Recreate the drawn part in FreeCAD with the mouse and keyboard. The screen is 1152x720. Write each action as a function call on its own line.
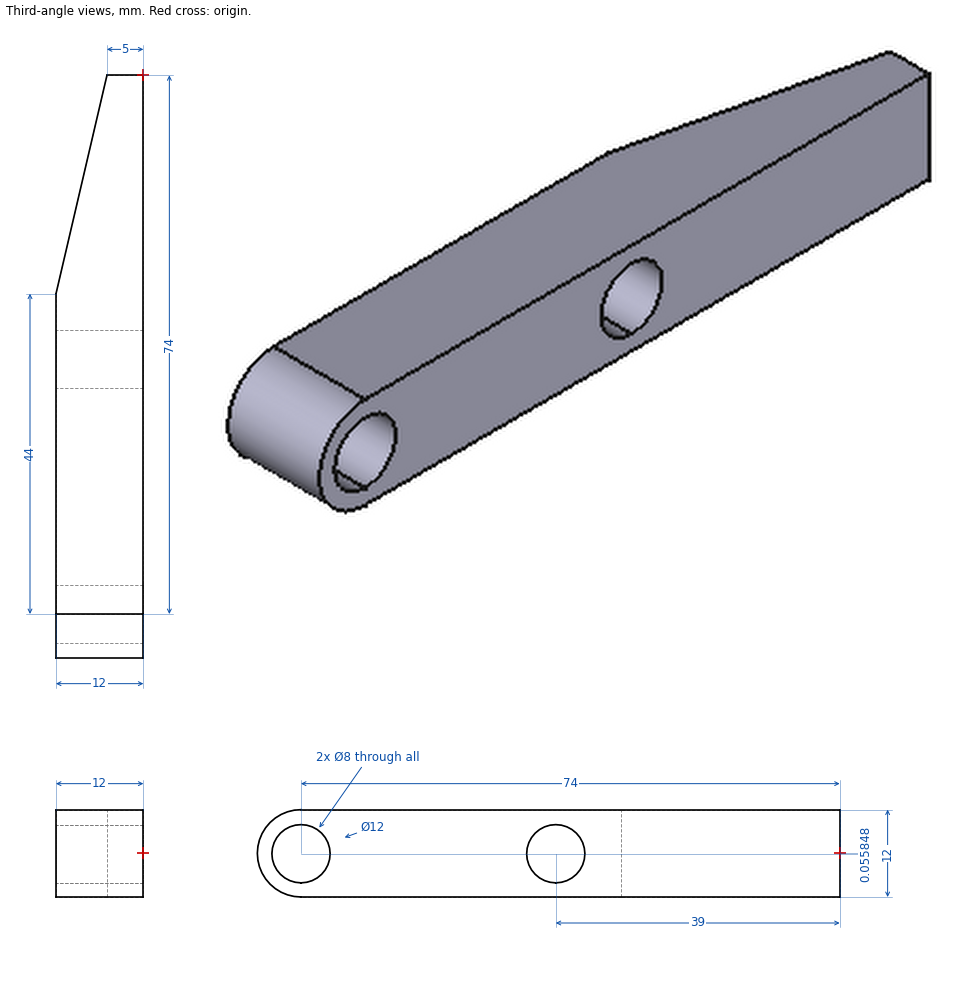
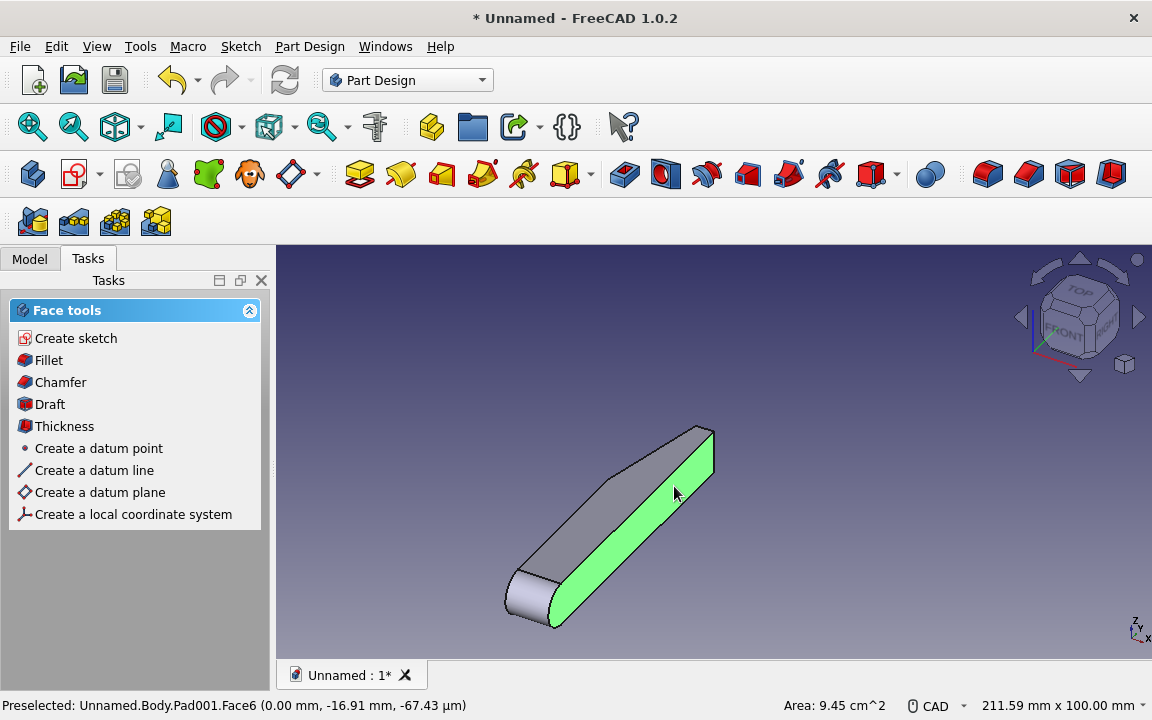
click(74, 174)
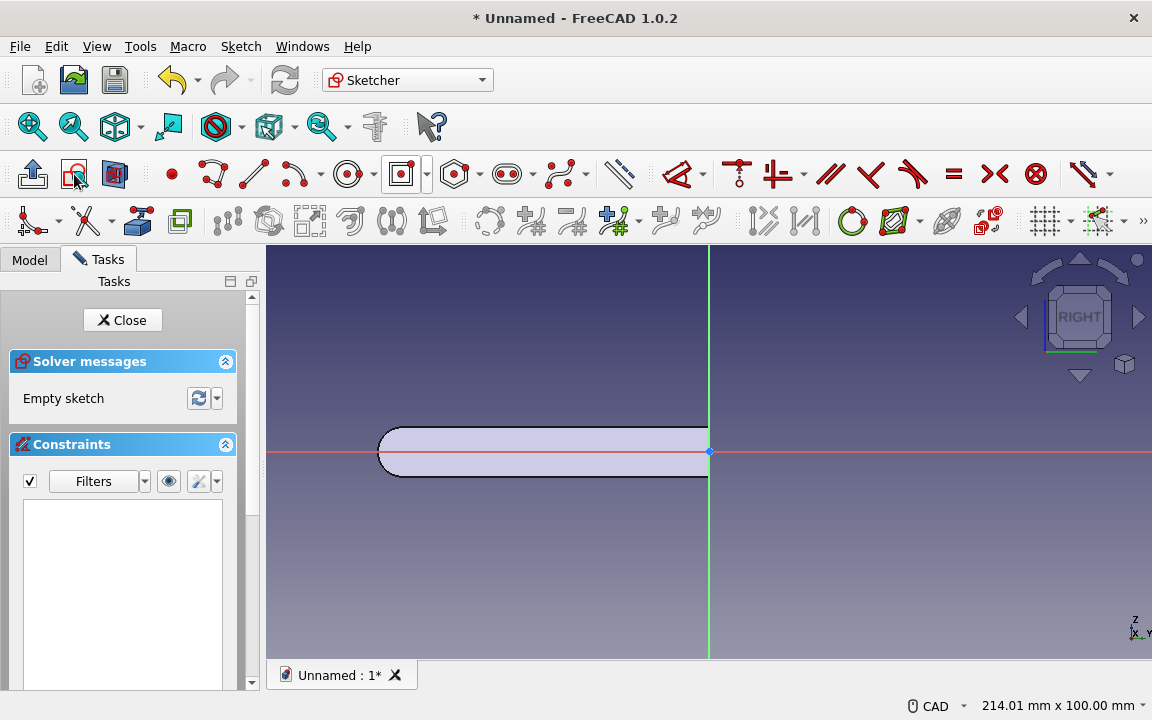
scroll(359, 453, up, 2)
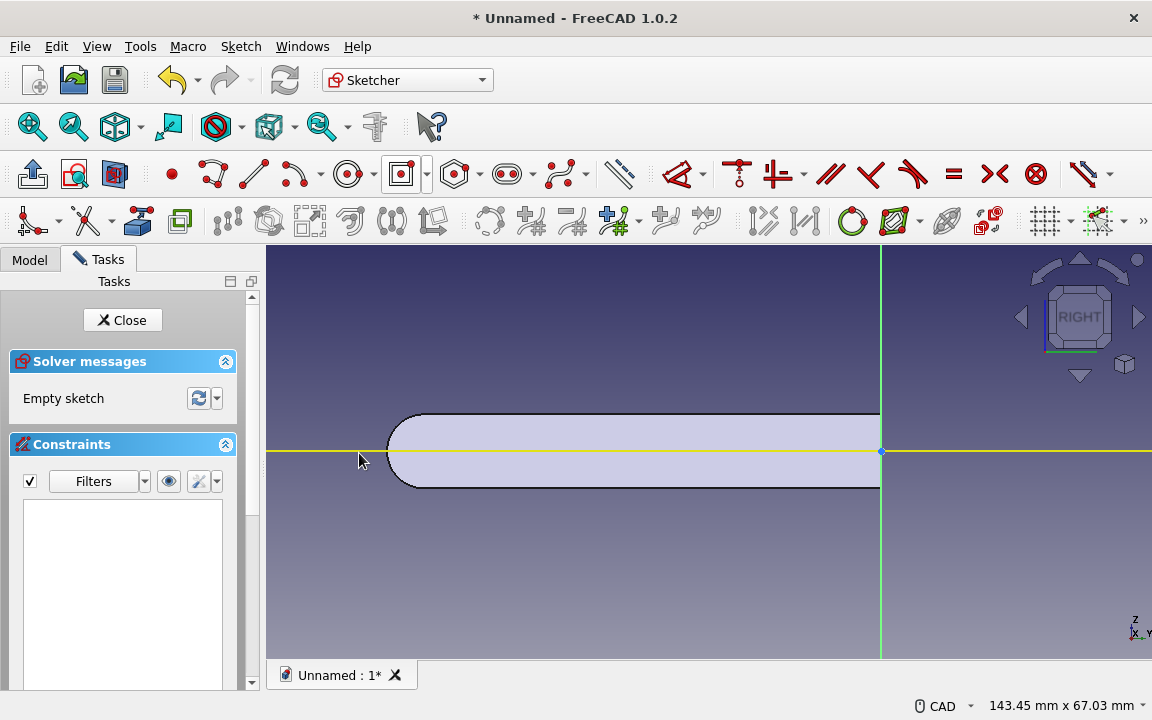
key(g)
key(c)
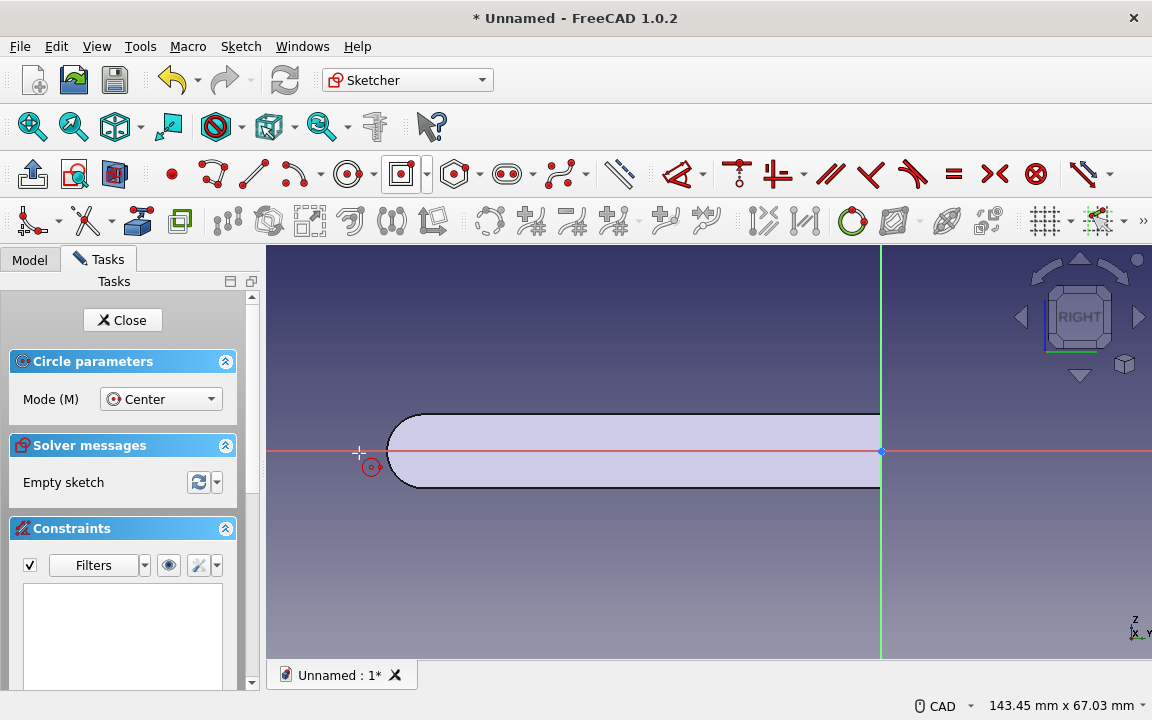
scroll(424, 452, up, 20)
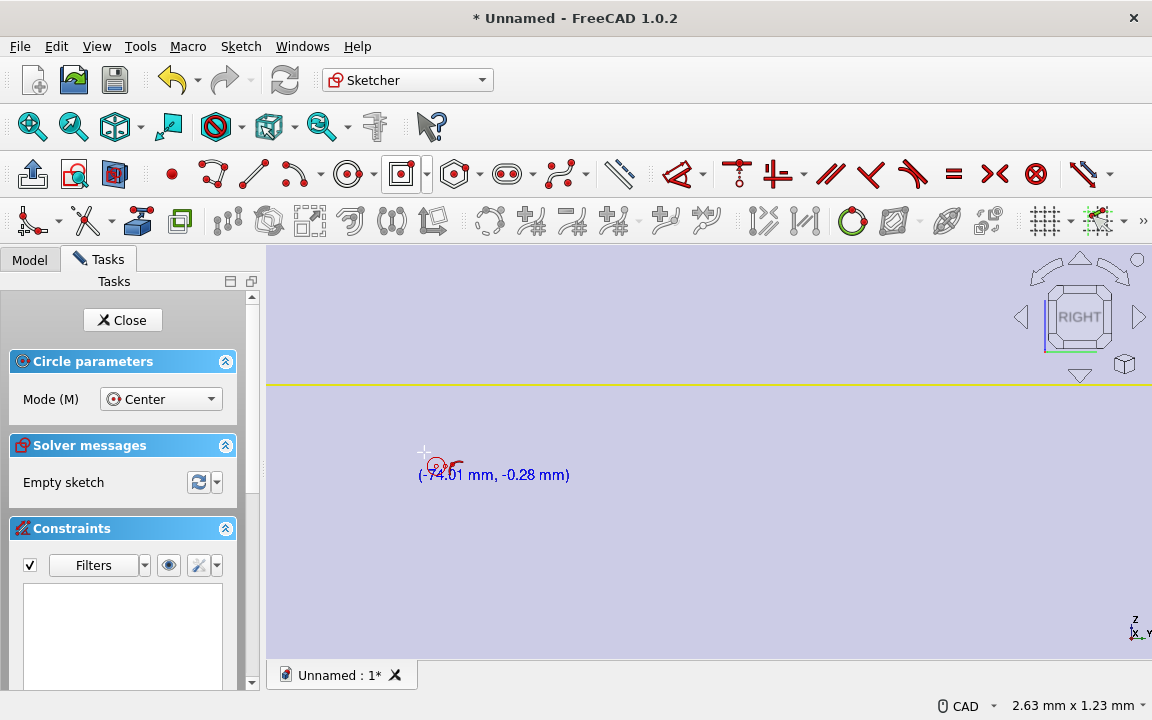
click(417, 404)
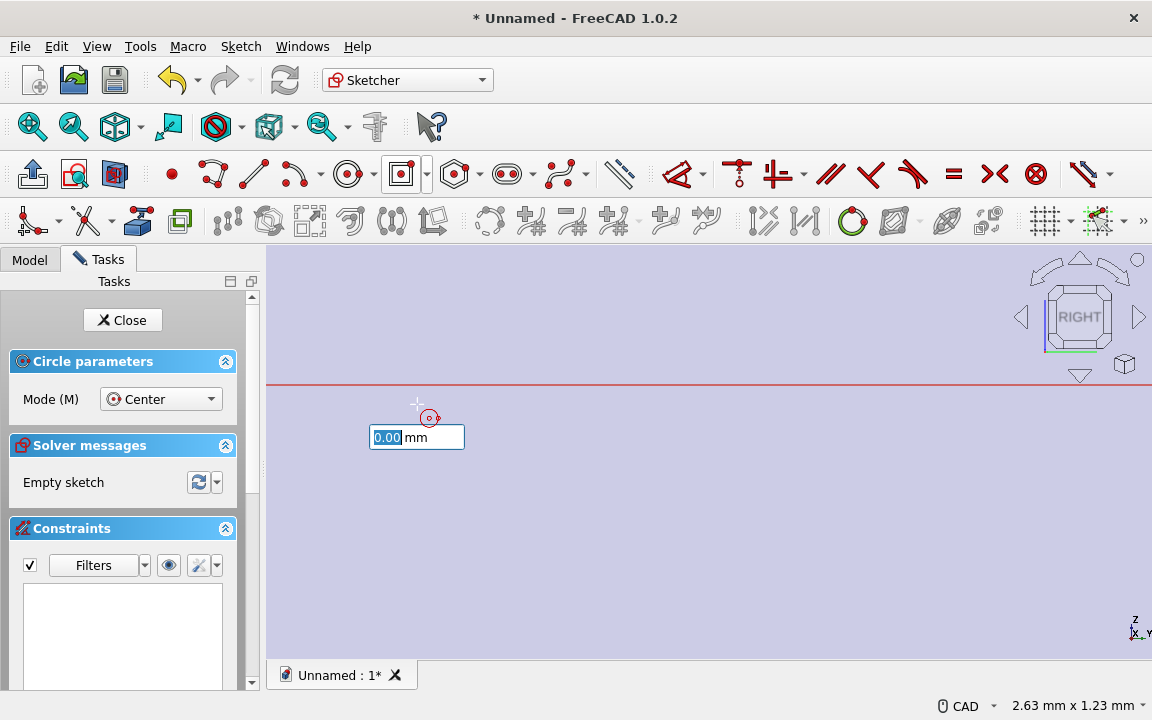
scroll(640, 452, down, 15)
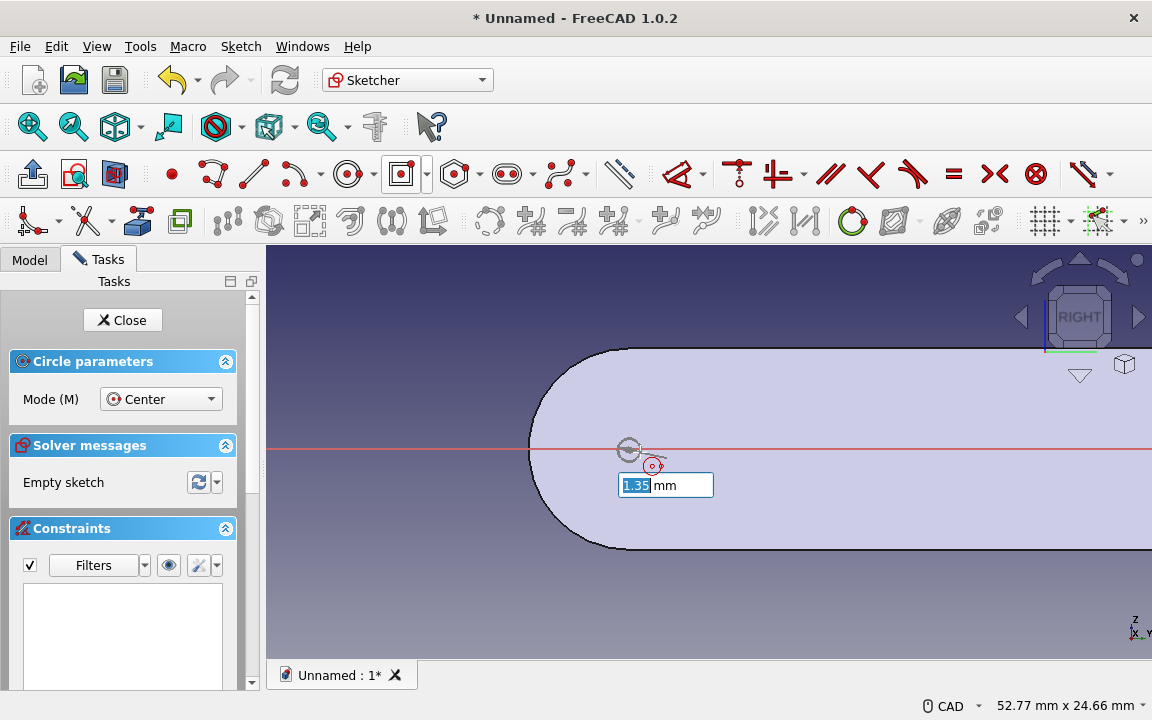
scroll(305, 453, down, 5)
move(442, 435)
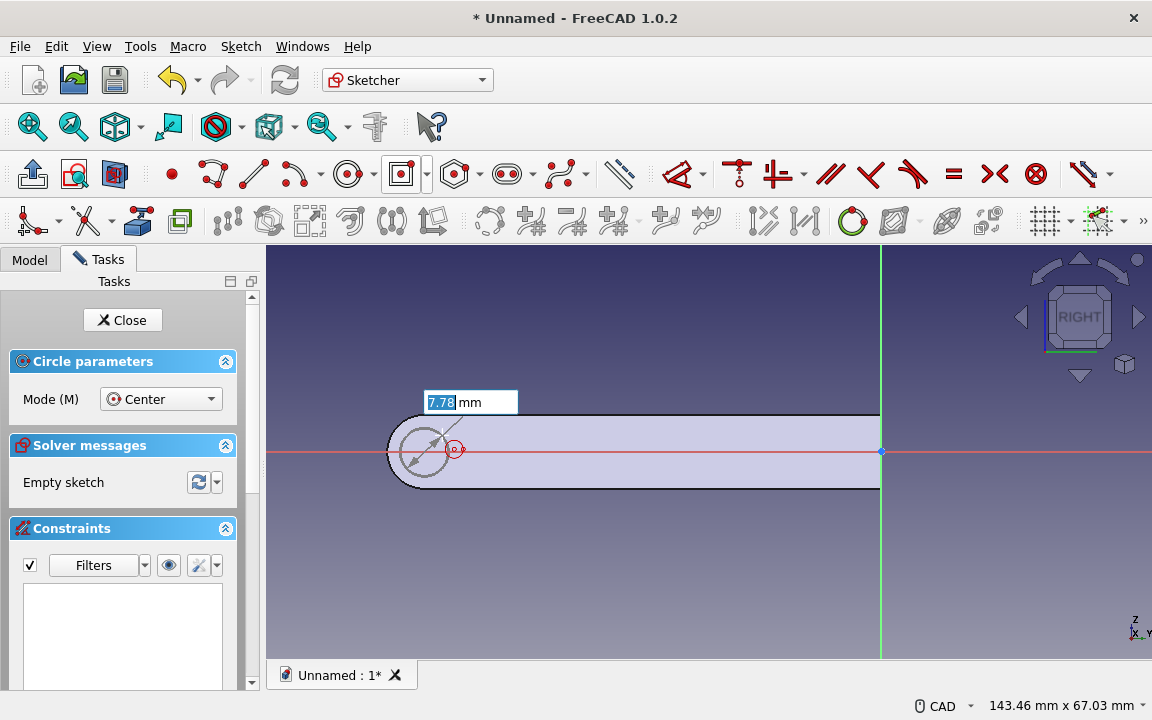
text(8)
key(Return)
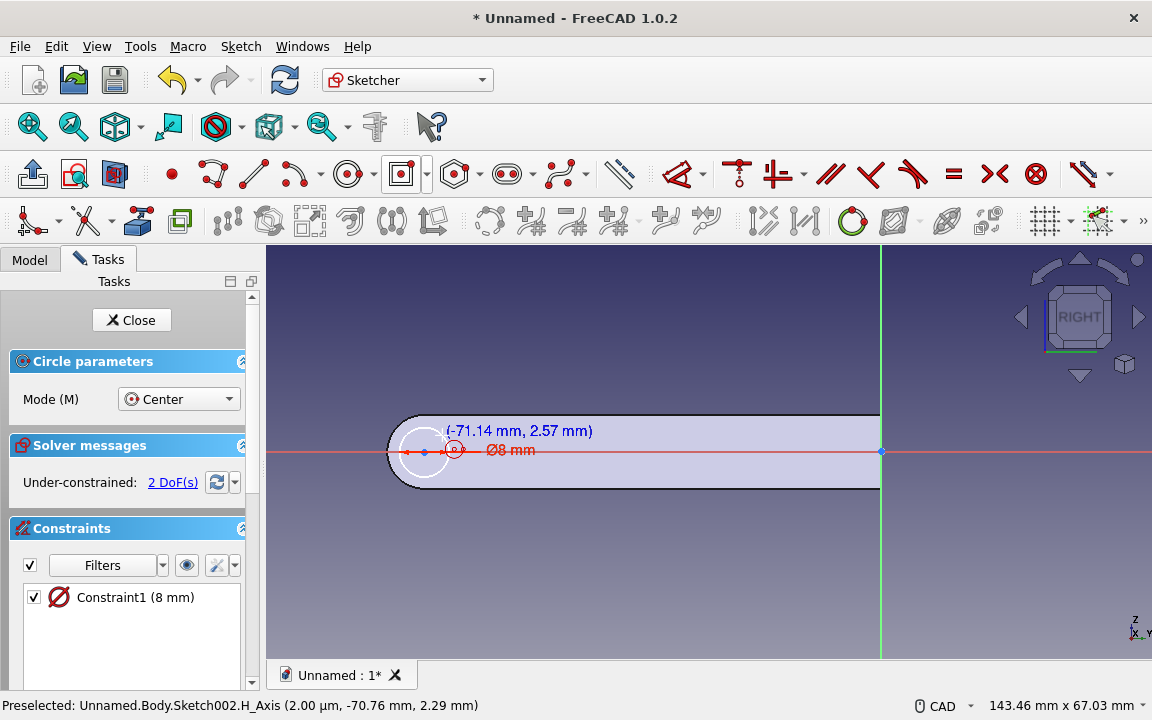
scroll(641, 452, up, 20)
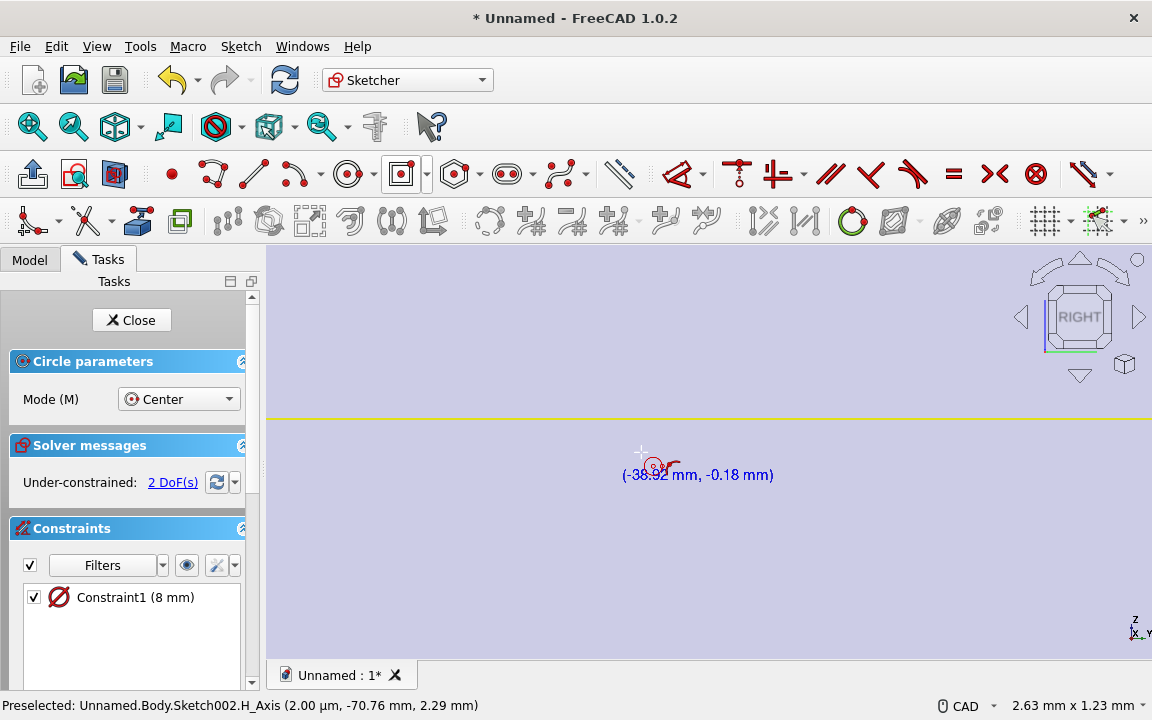
click(591, 438)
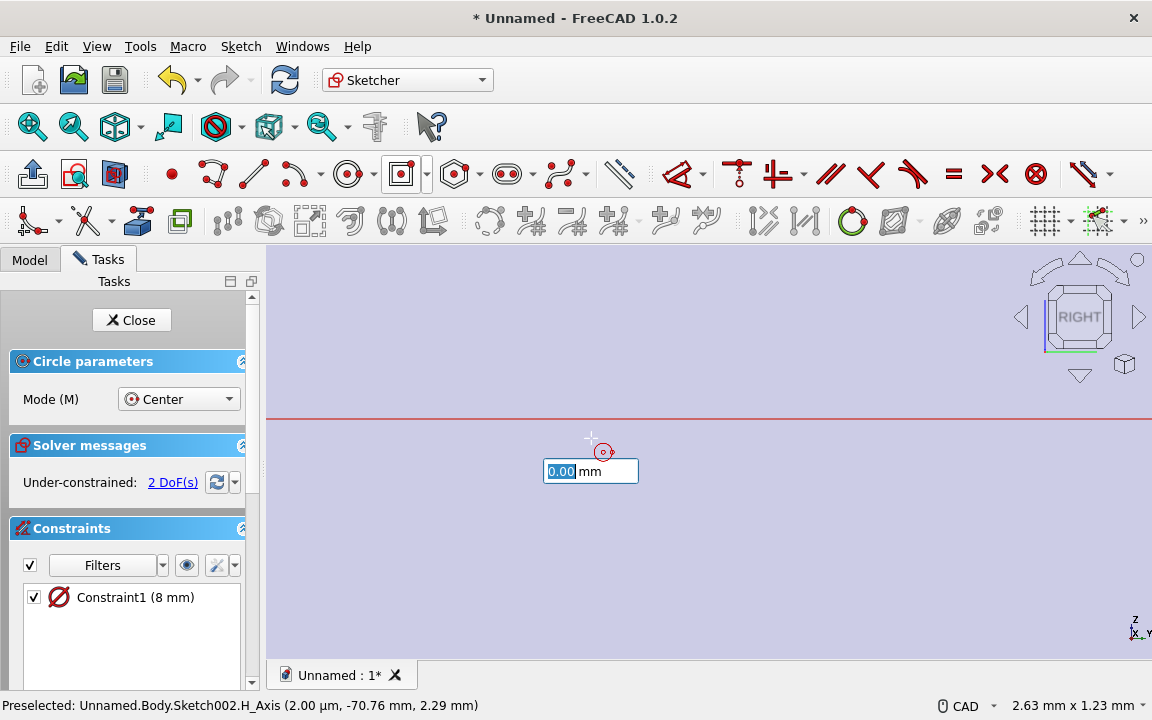
scroll(640, 452, down, 15)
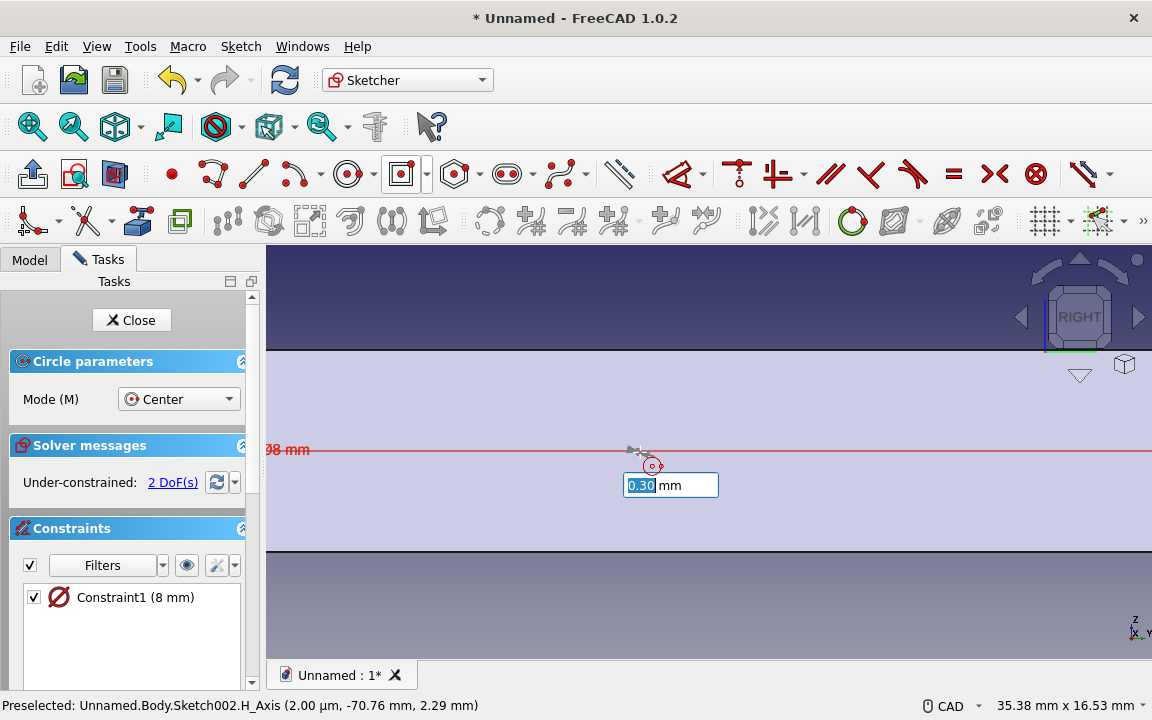
scroll(642, 452, down, 5)
move(658, 435)